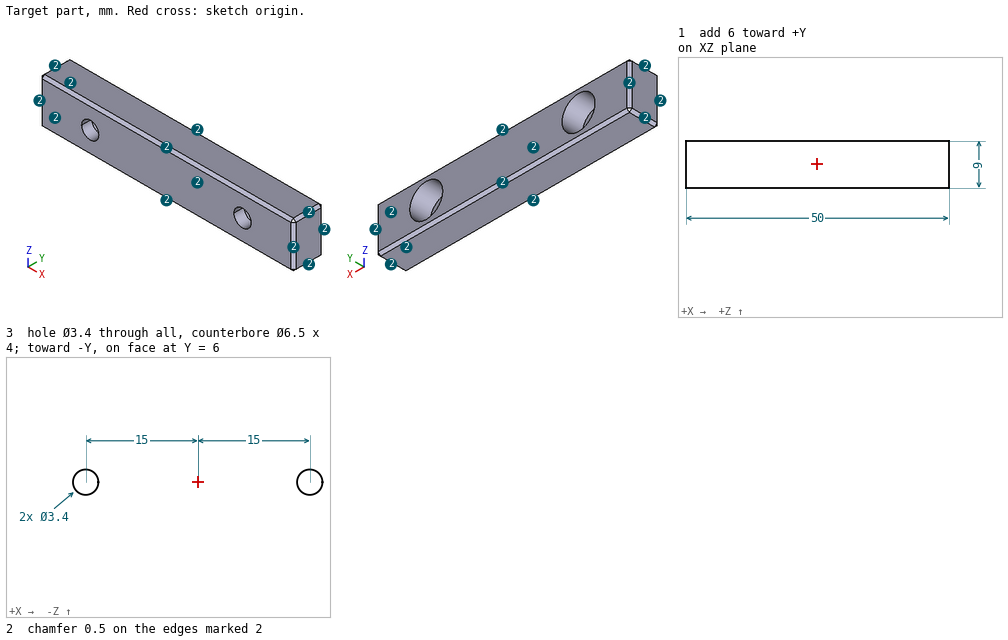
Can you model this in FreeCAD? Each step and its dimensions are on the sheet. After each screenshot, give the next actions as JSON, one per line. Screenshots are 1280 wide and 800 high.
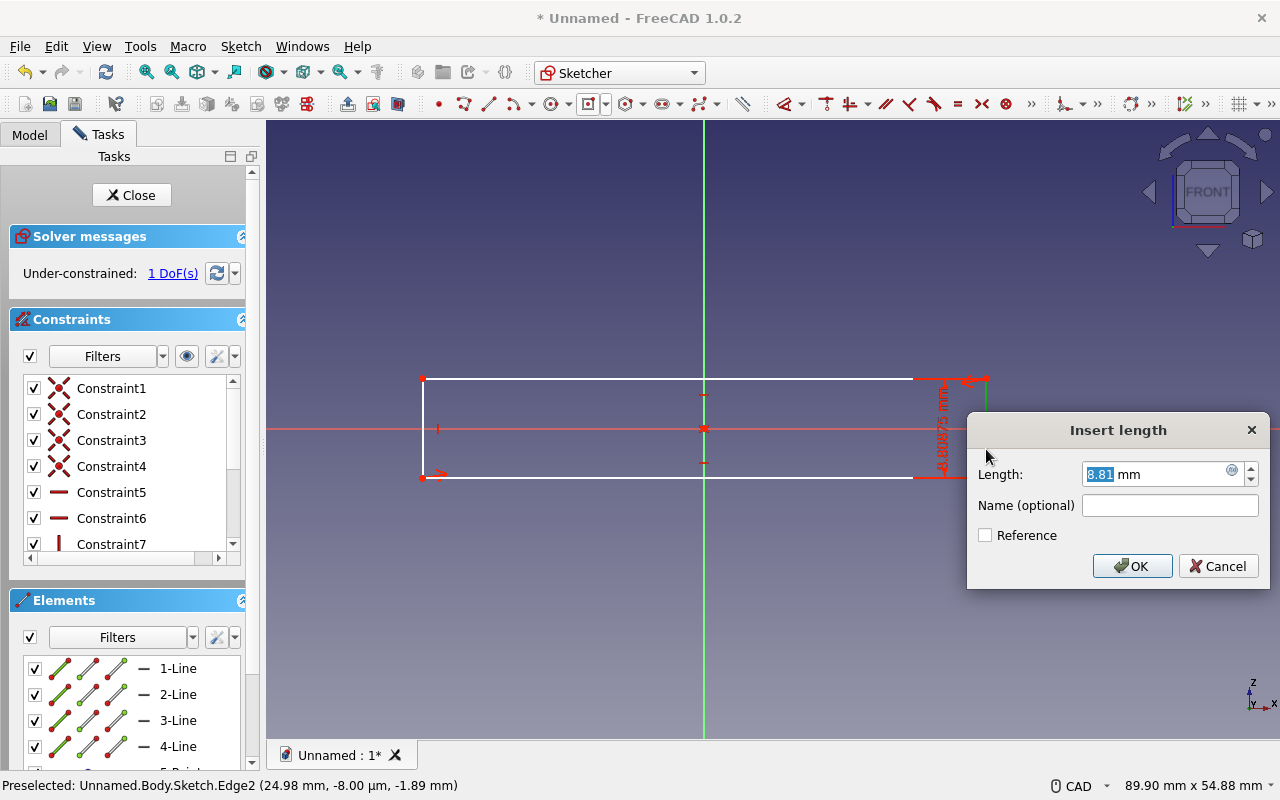
{"action": "type", "text": "9"}
{"action": "key", "text": "Return"}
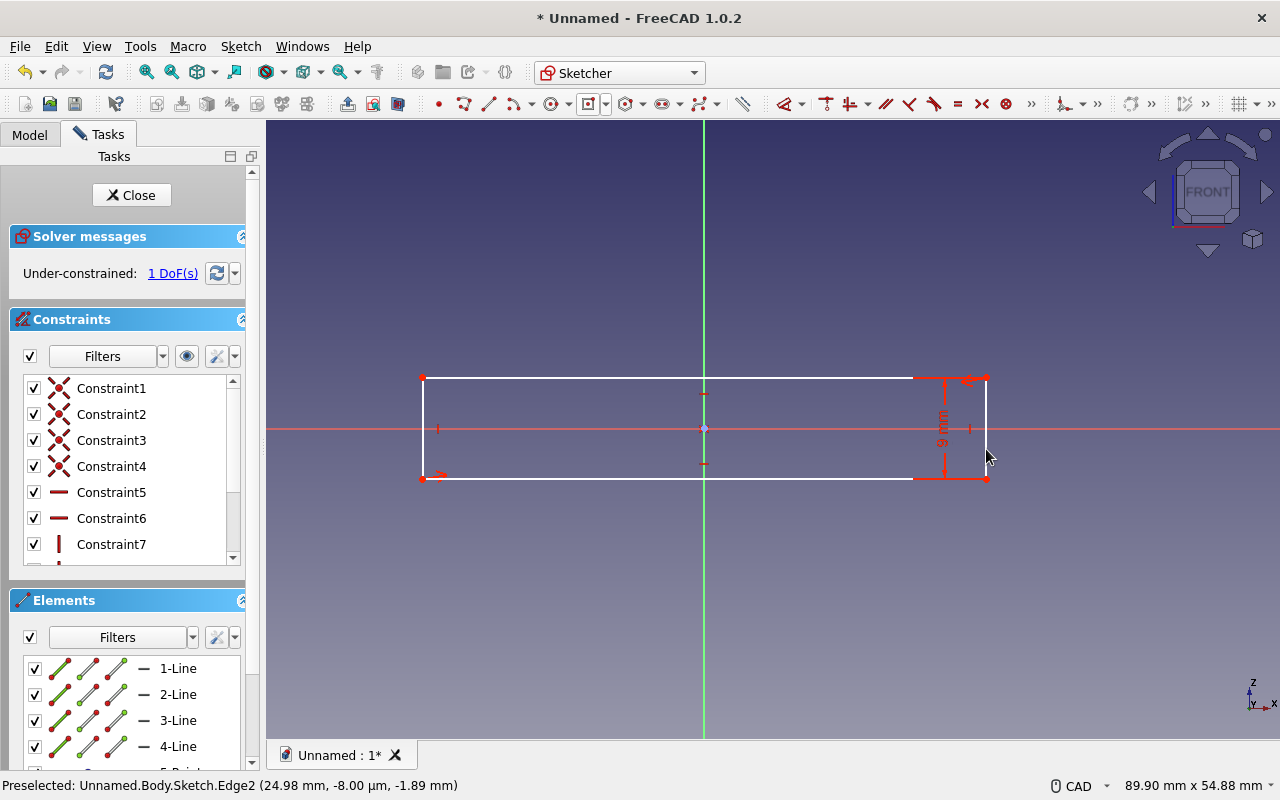
{"action": "left_click", "coordinate": [592, 479]}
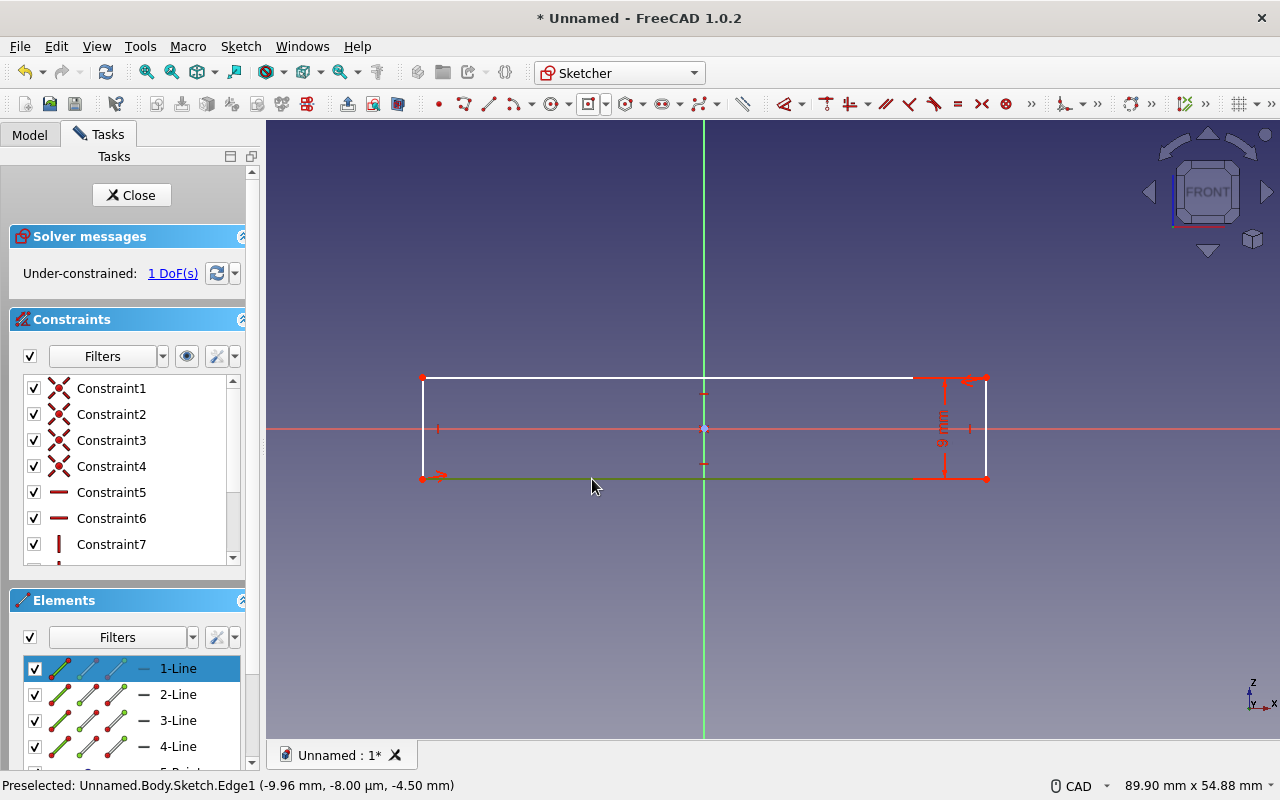
{"action": "left_click", "coordinate": [802, 104]}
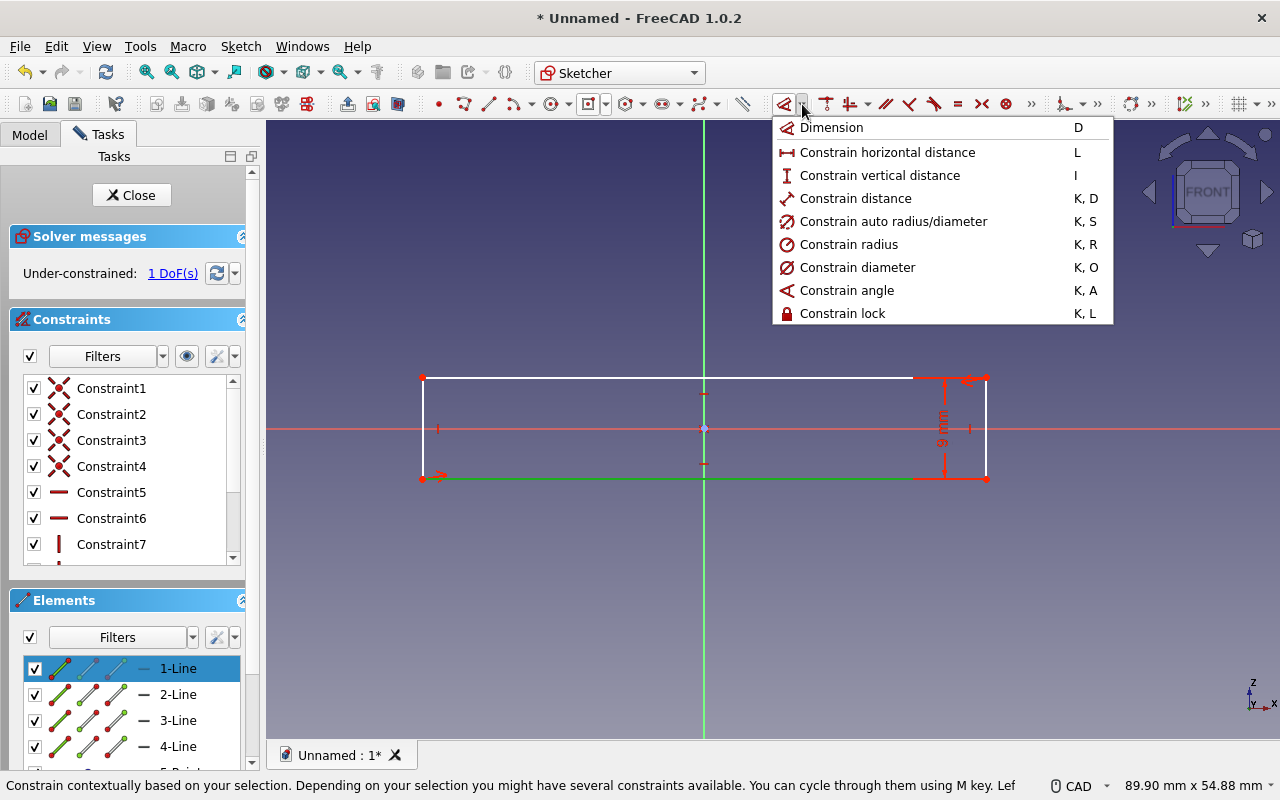
{"action": "left_click", "coordinate": [943, 152]}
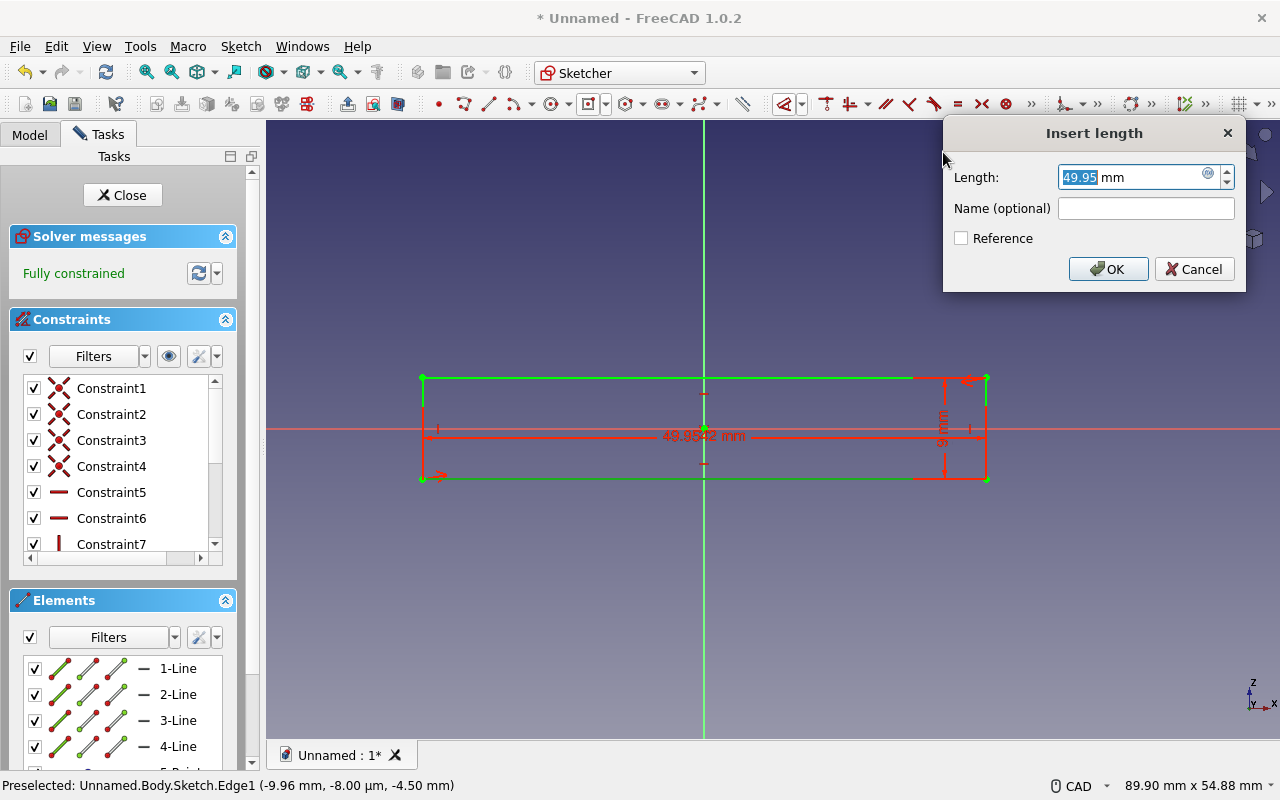
{"action": "type", "text": "50"}
{"action": "key", "text": "Return"}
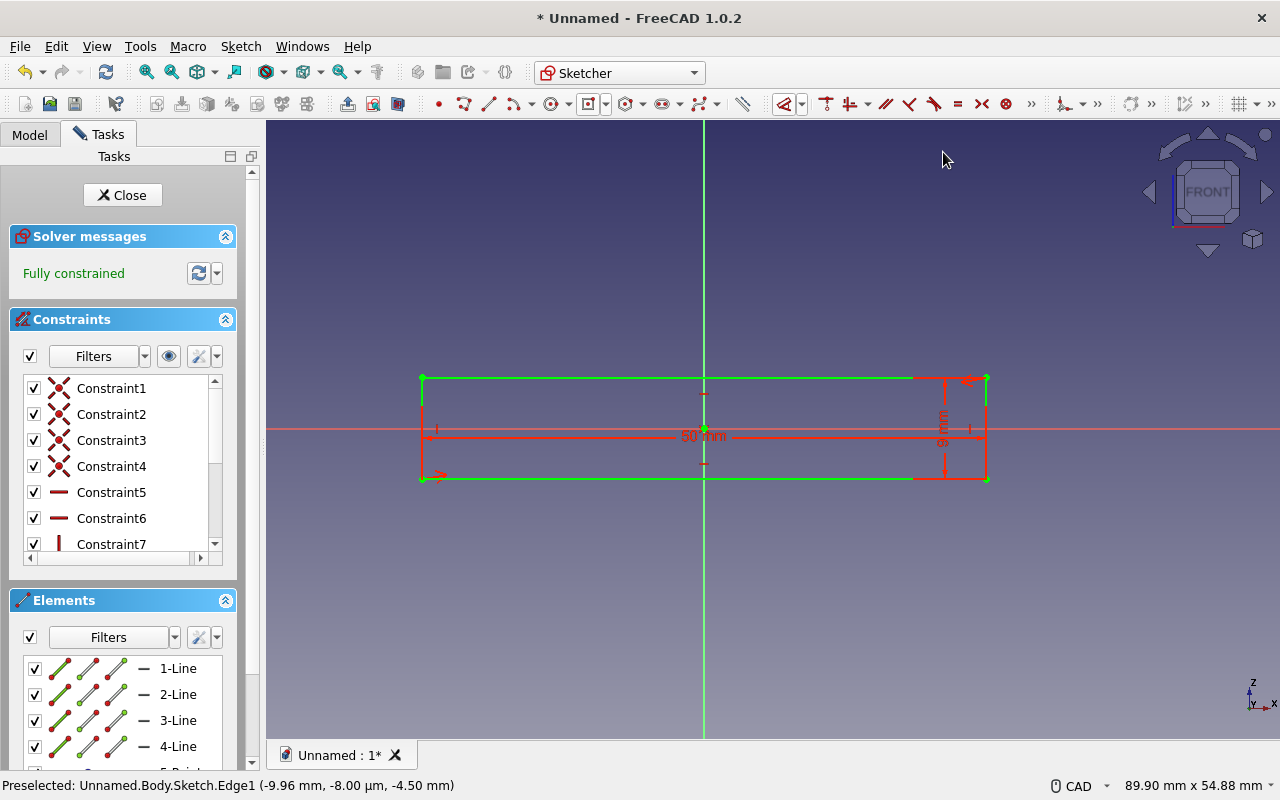
{"action": "left_click", "coordinate": [123, 195]}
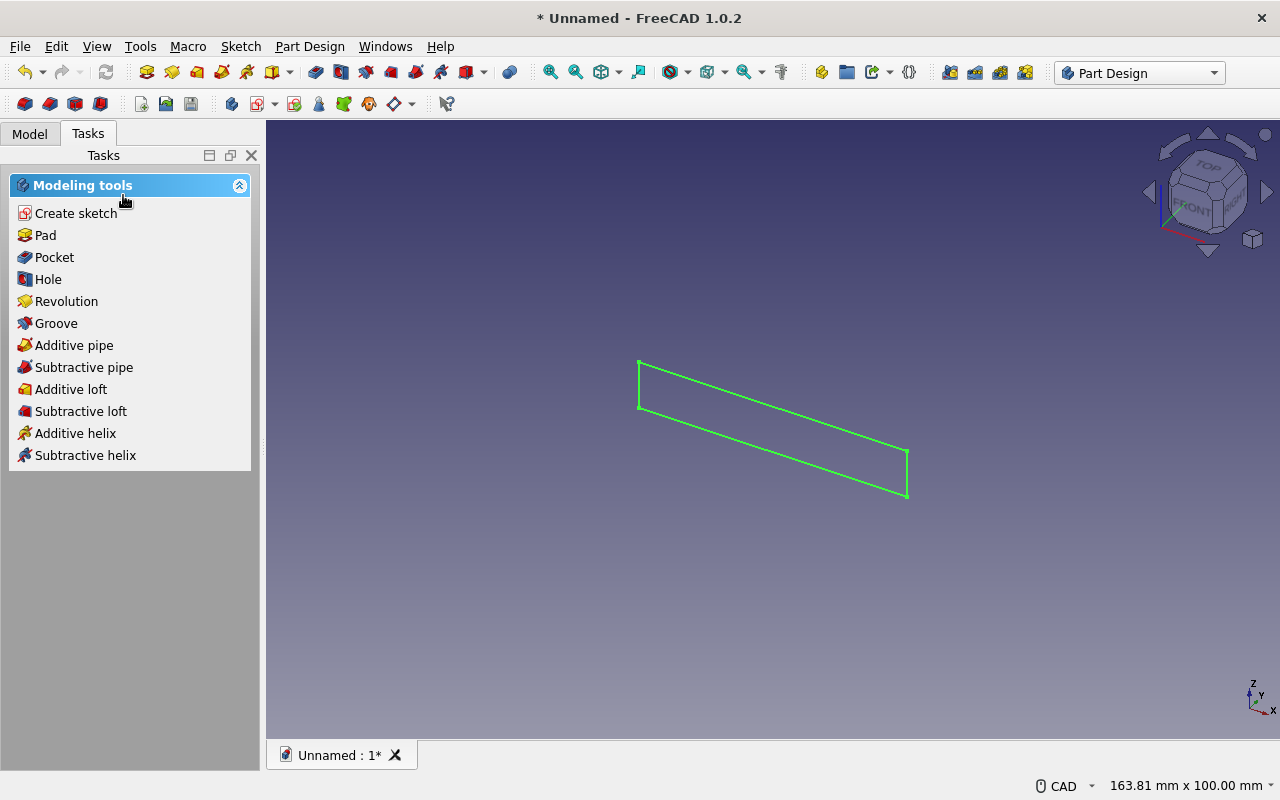
{"action": "left_click", "coordinate": [147, 72]}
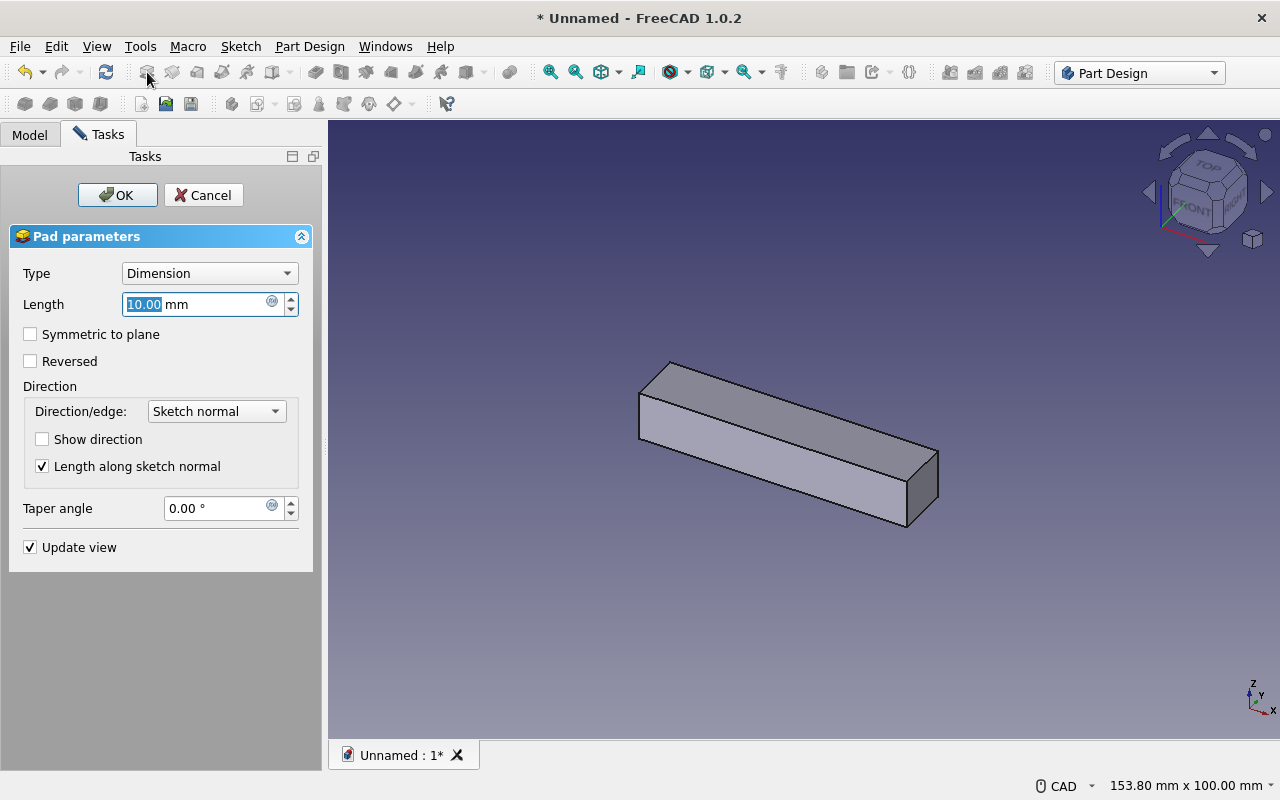
{"action": "type", "text": "6"}
{"action": "key", "text": "Tab"}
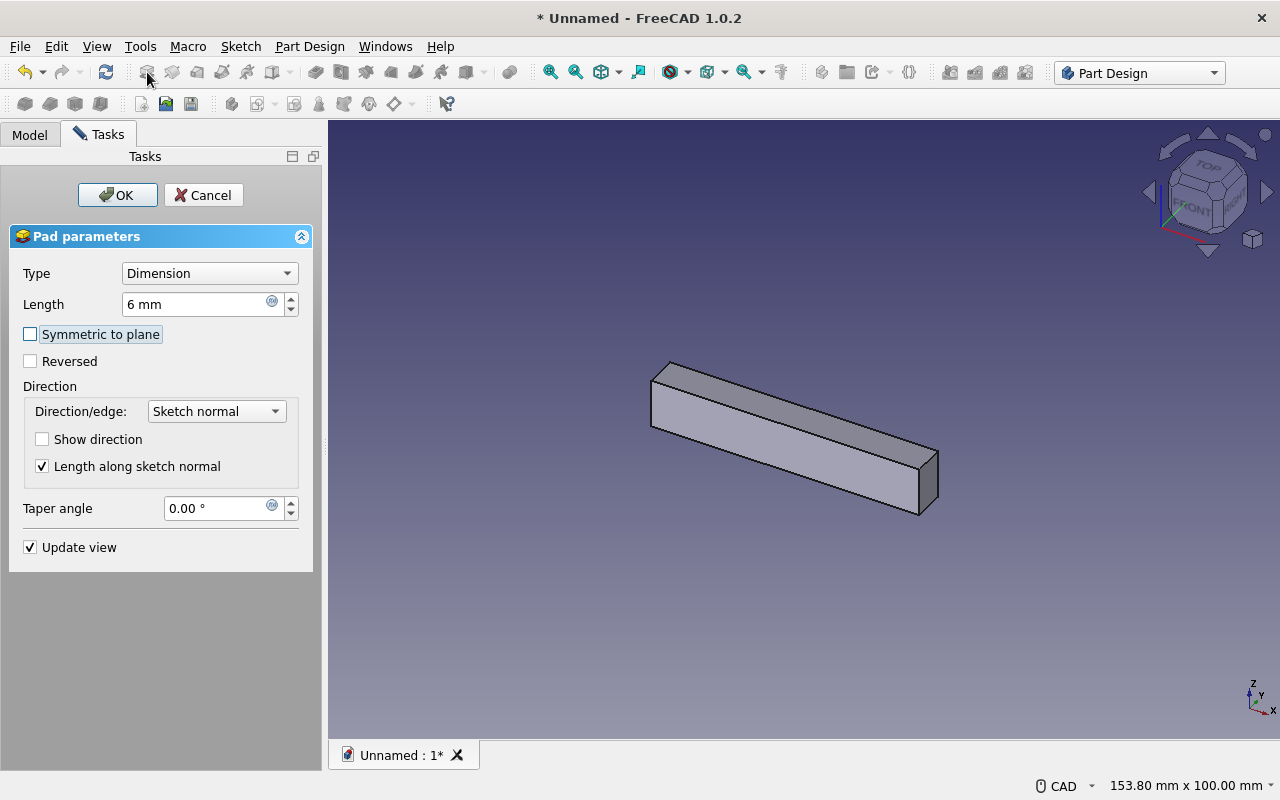
{"action": "left_click", "coordinate": [31, 361]}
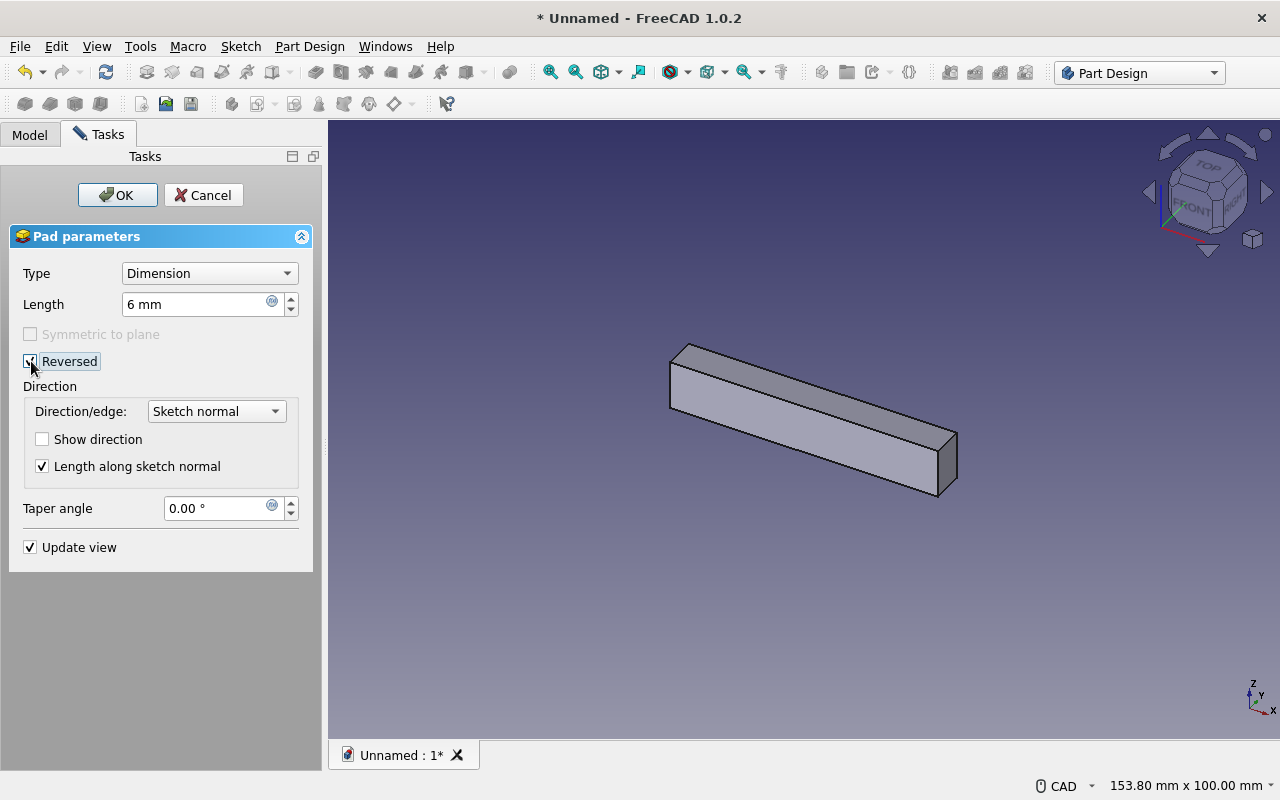
{"action": "left_click", "coordinate": [118, 195]}